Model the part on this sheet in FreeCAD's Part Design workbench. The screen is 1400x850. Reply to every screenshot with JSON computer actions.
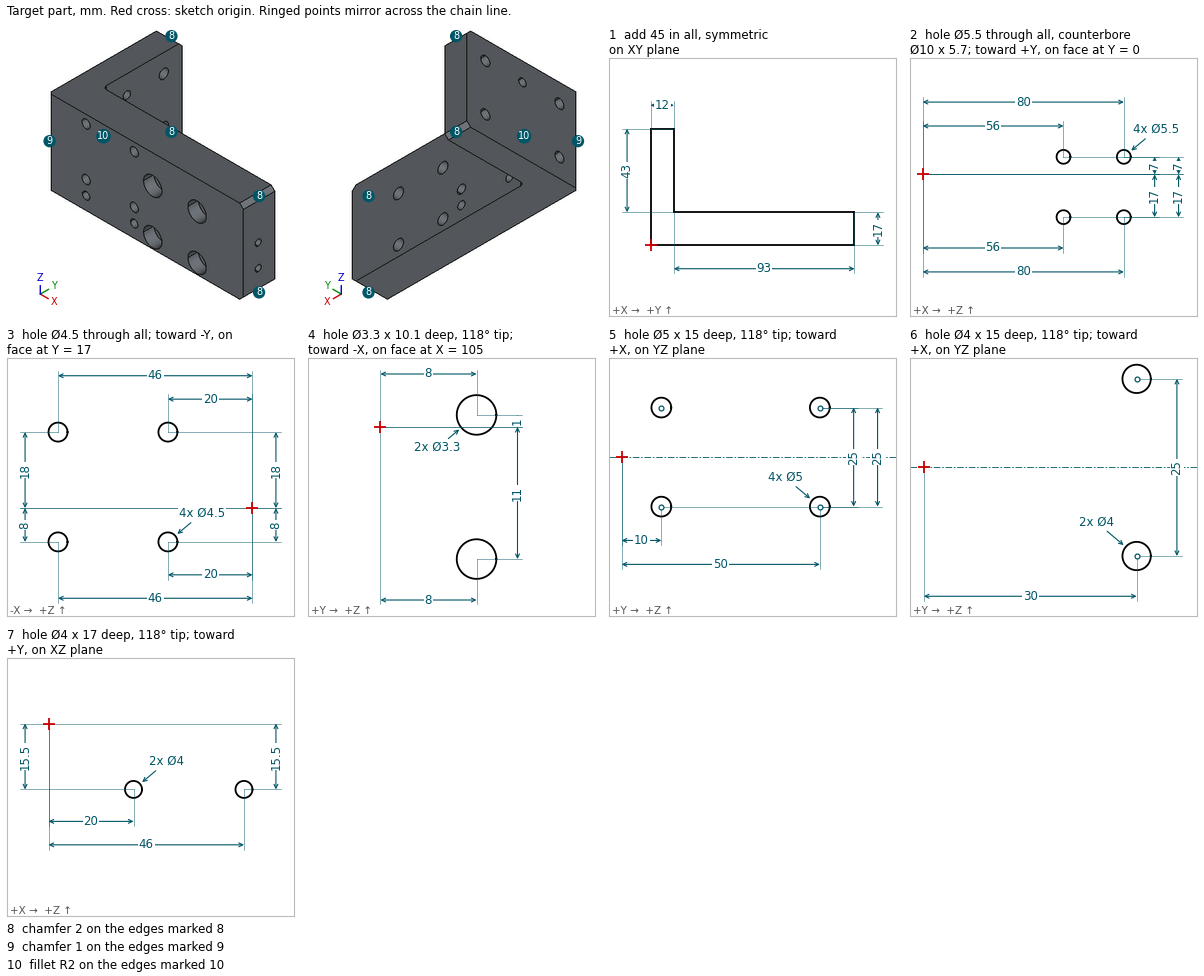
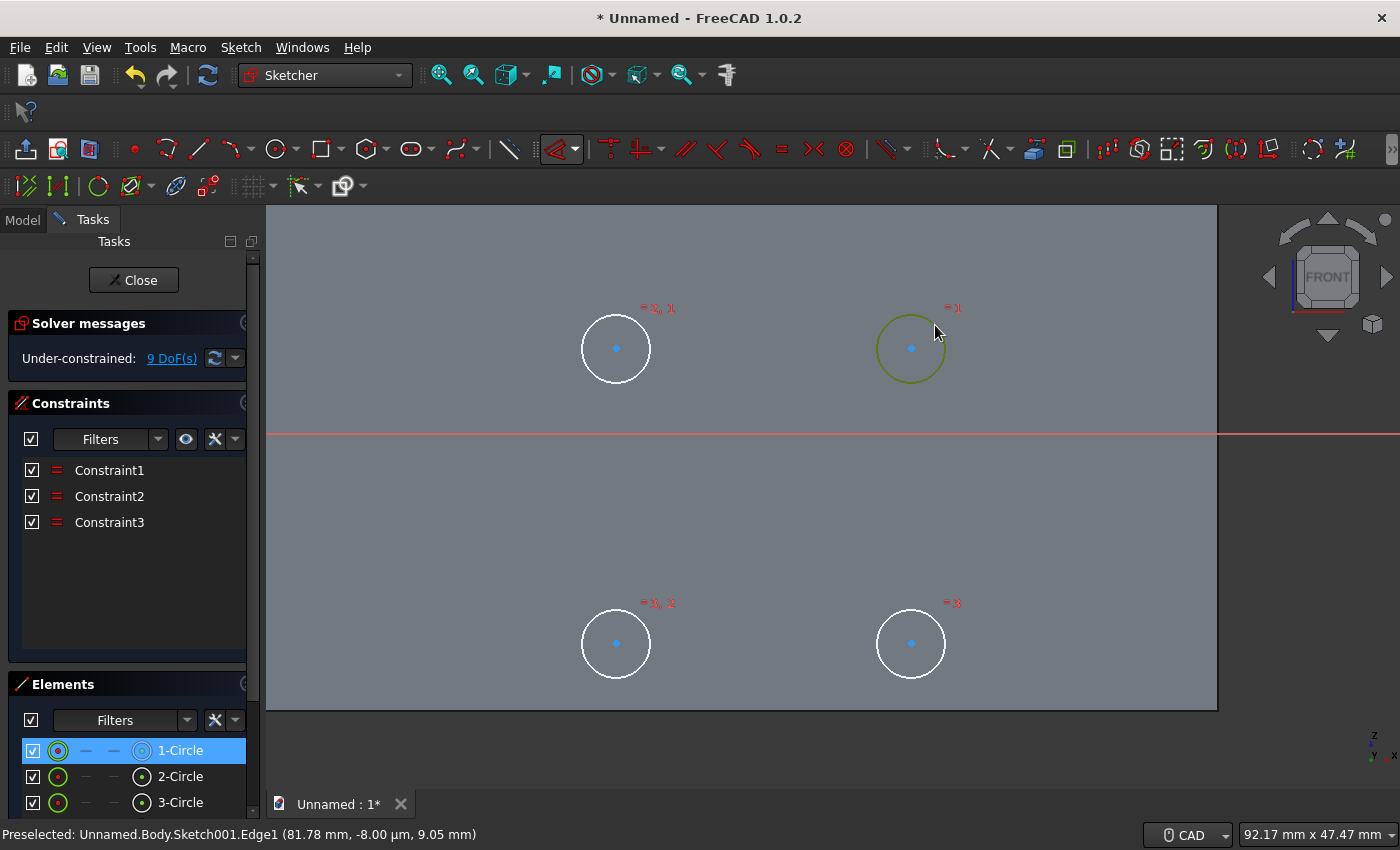
{"action": "key", "text": "k o"}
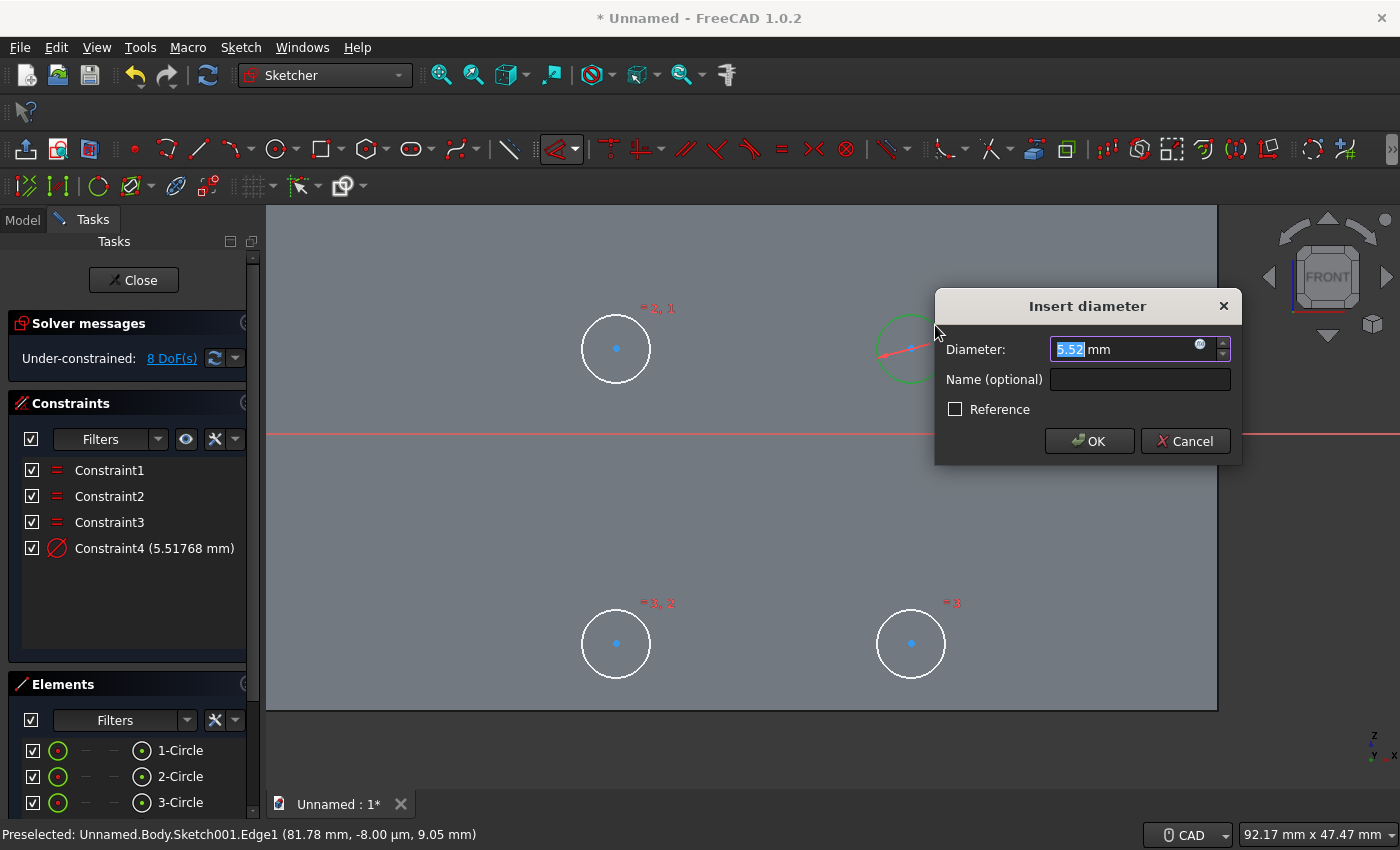
{"action": "type", "text": "5.5"}
{"action": "key", "text": "Return"}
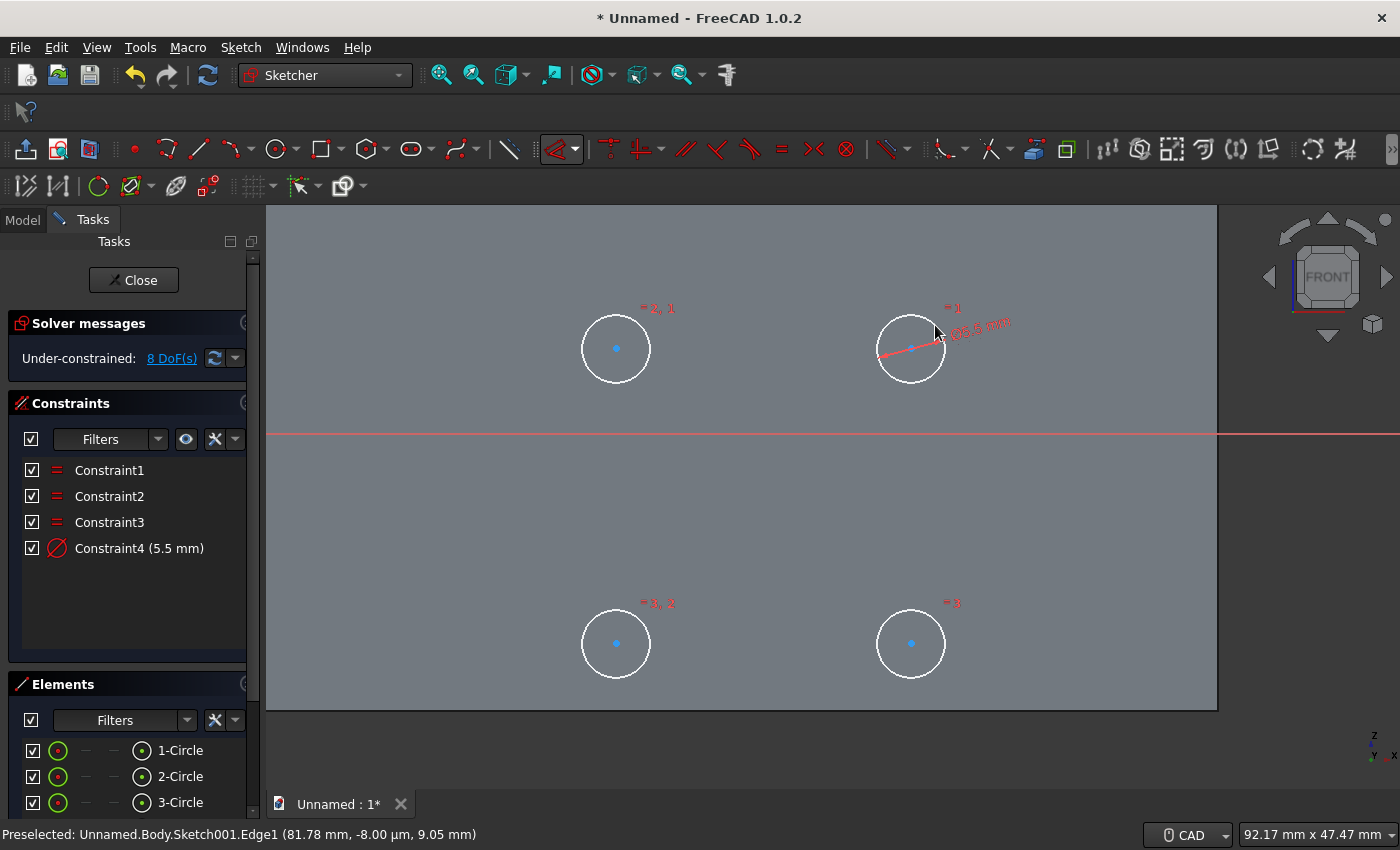
{"action": "left_click", "coordinate": [911, 349]}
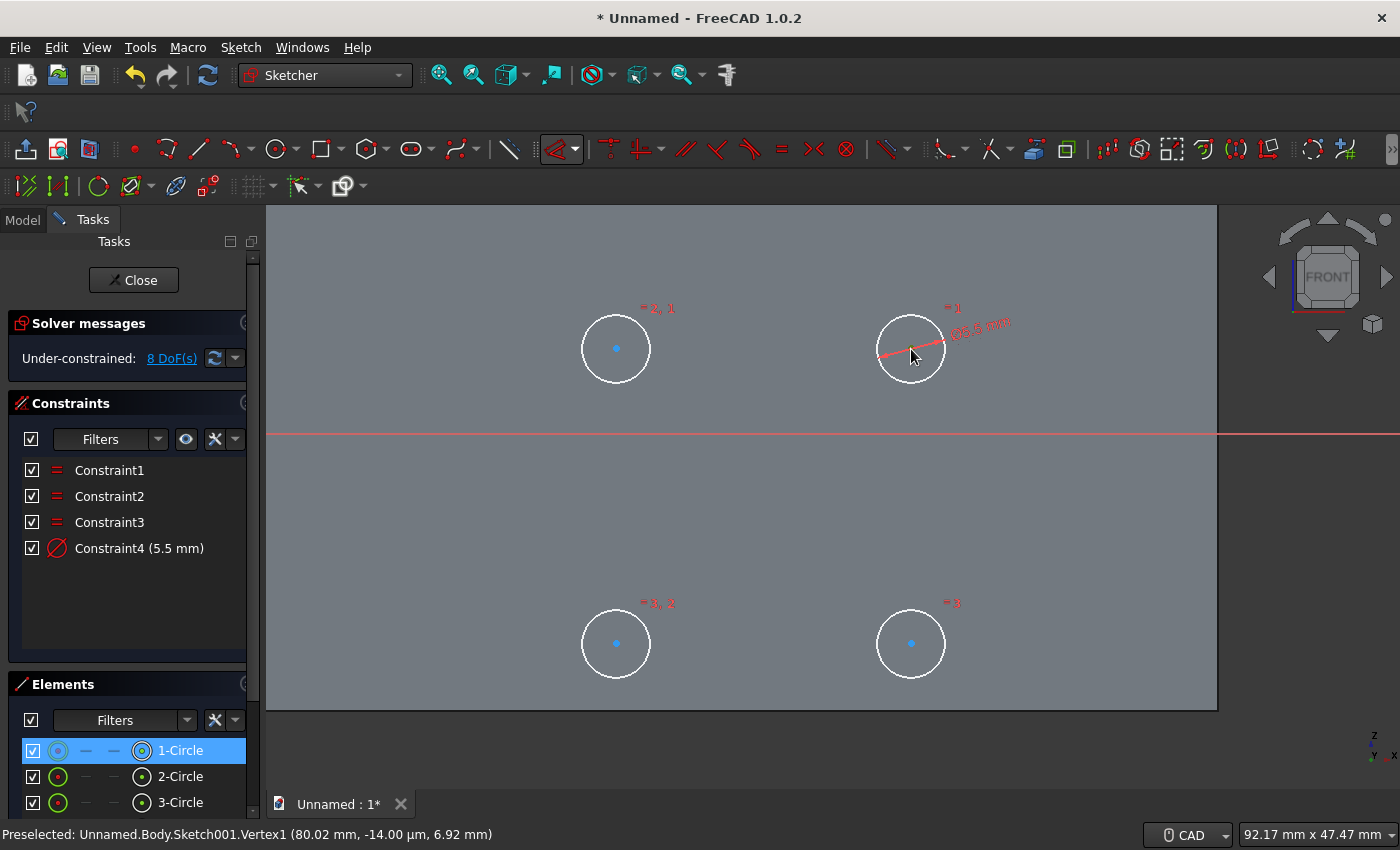
{"action": "key", "text": "i"}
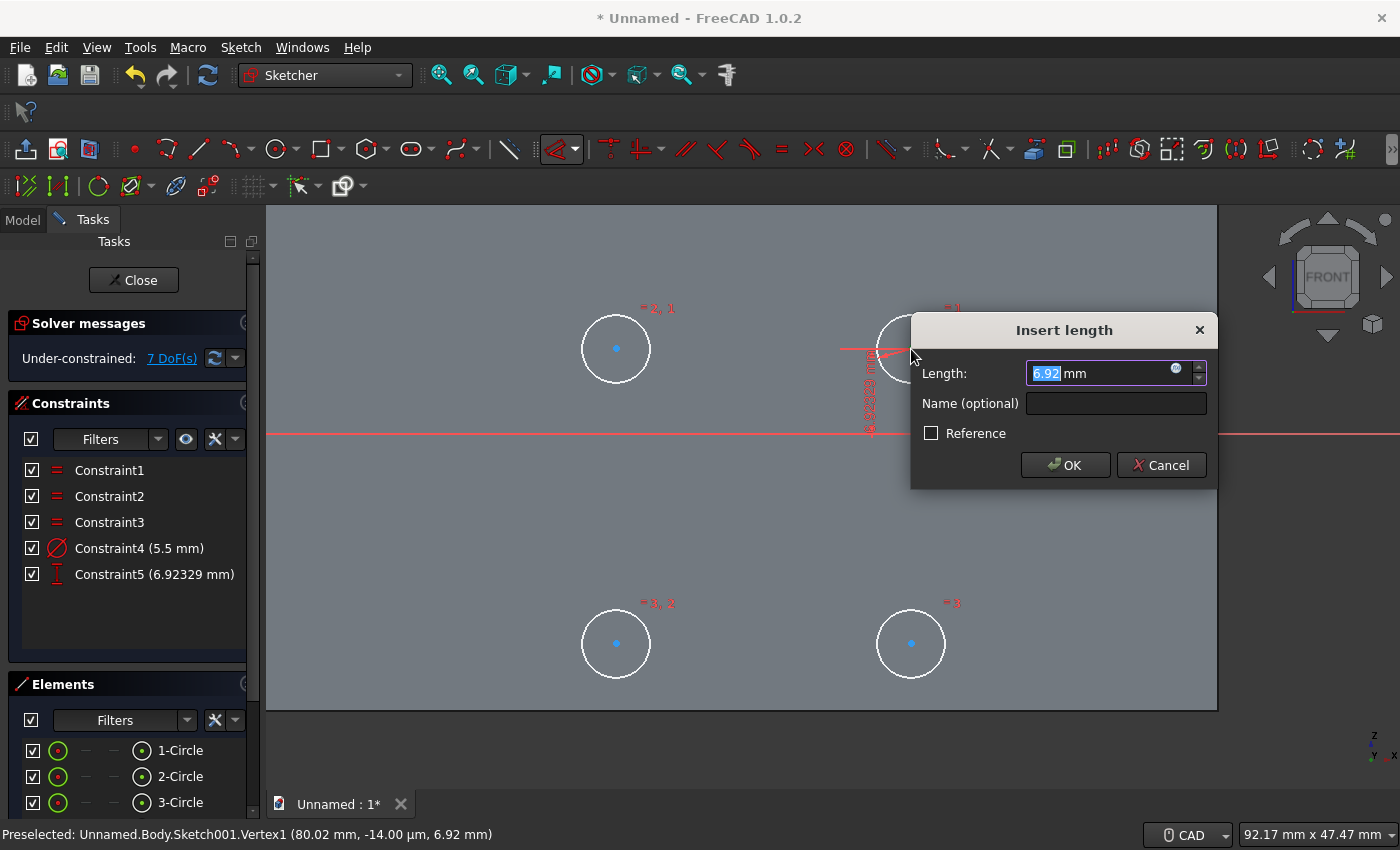
{"action": "type", "text": "7"}
{"action": "key", "text": "Return"}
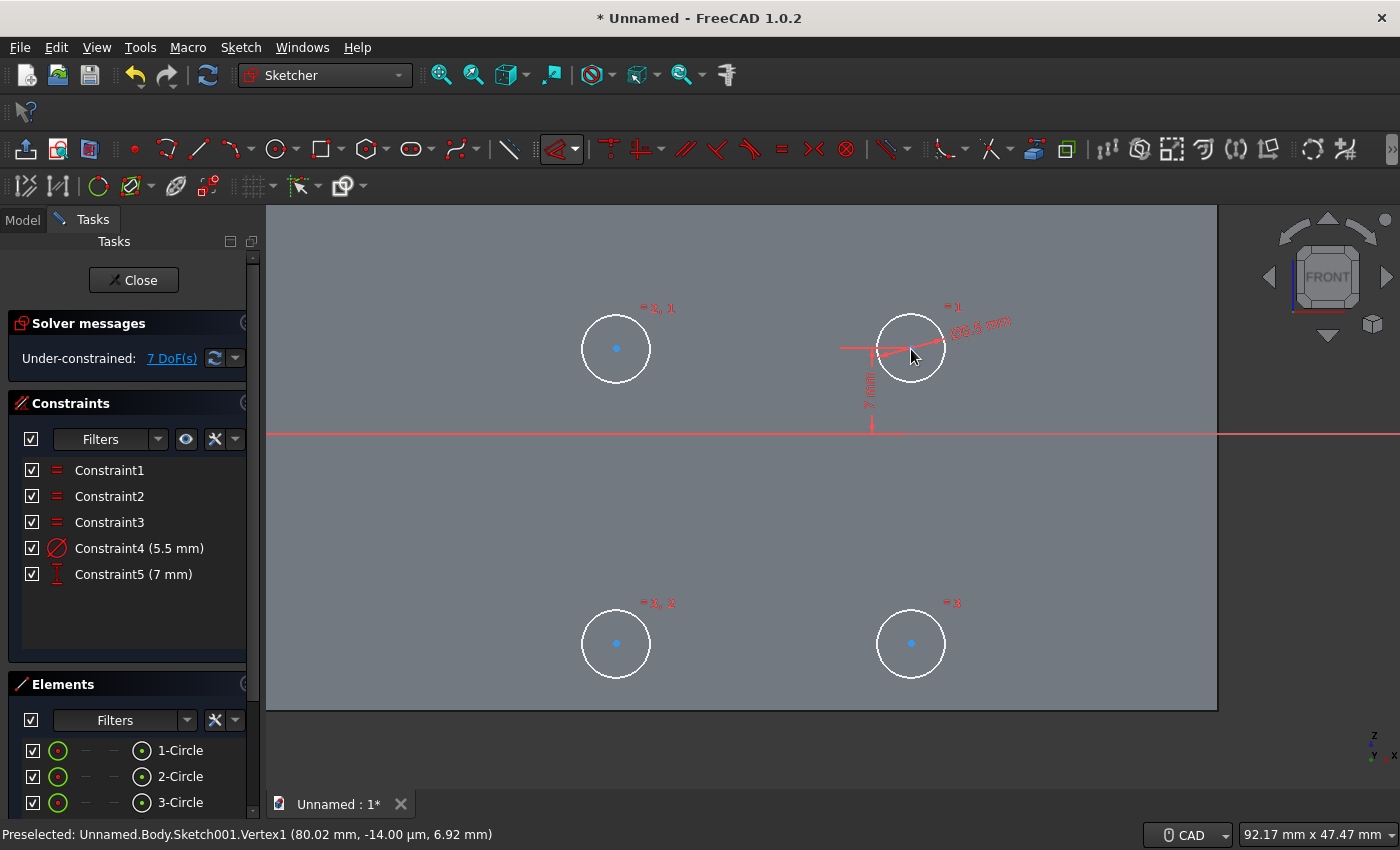
{"action": "left_click", "coordinate": [616, 349]}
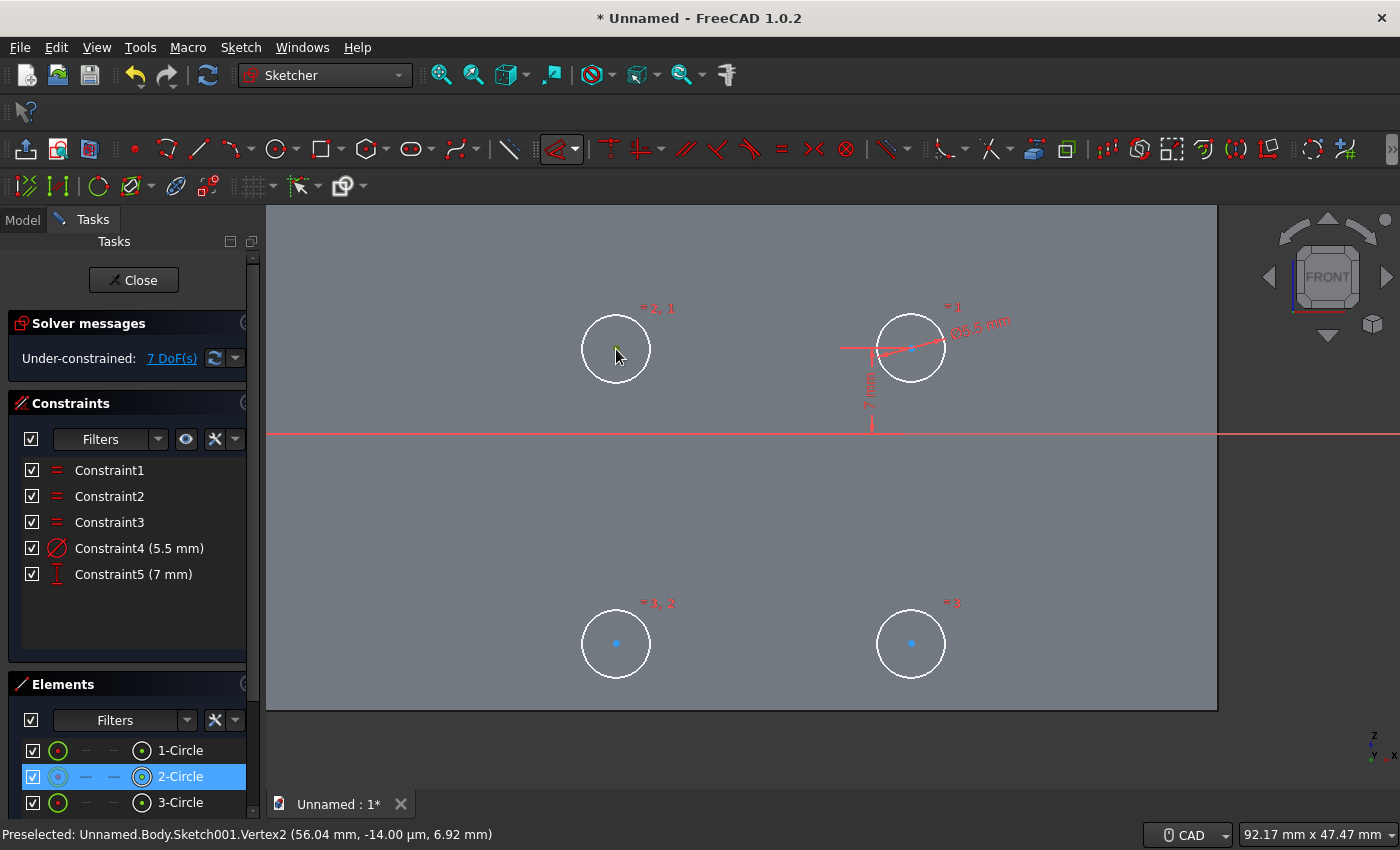
{"action": "left_click", "coordinate": [578, 150]}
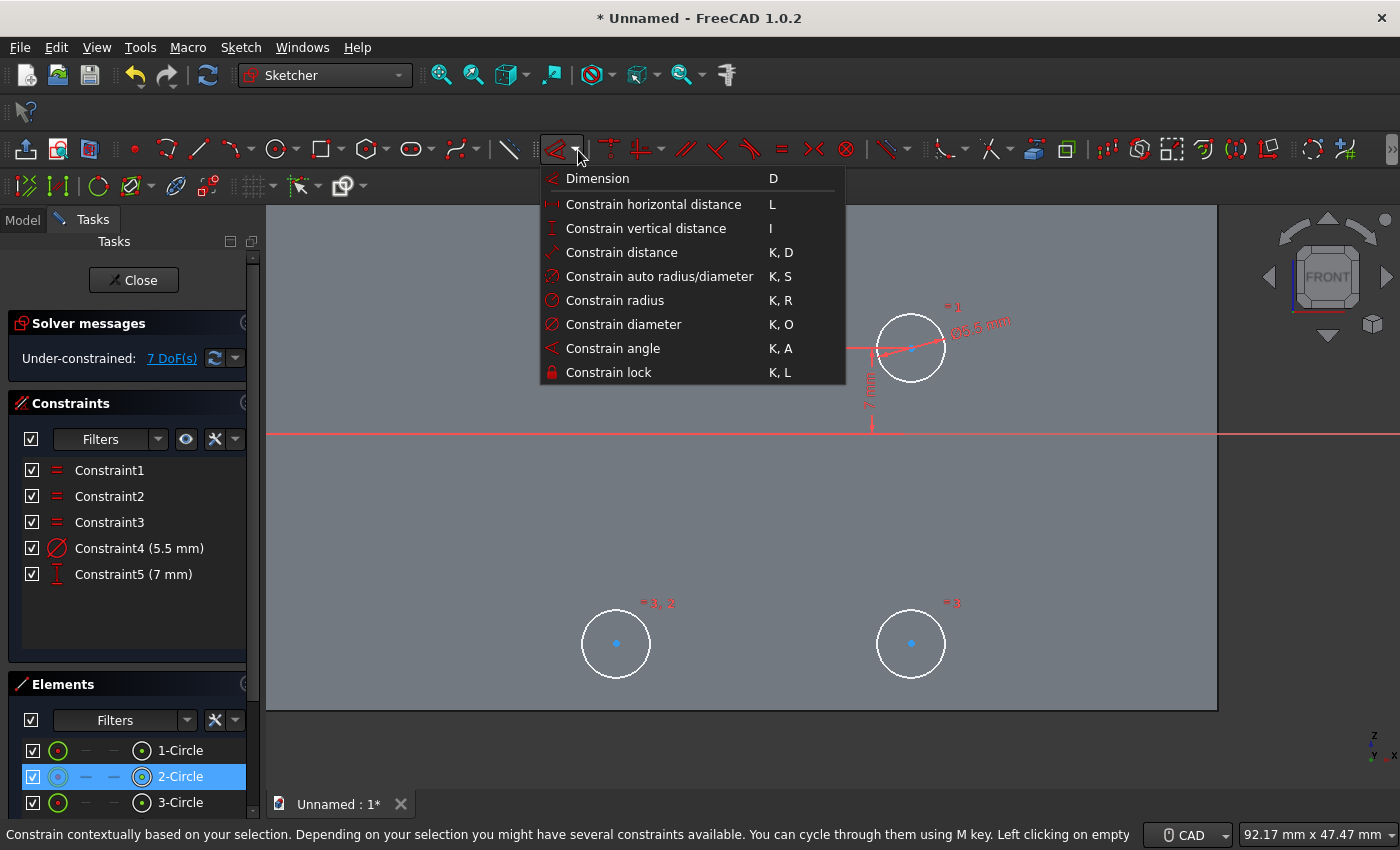
{"action": "left_click", "coordinate": [693, 228]}